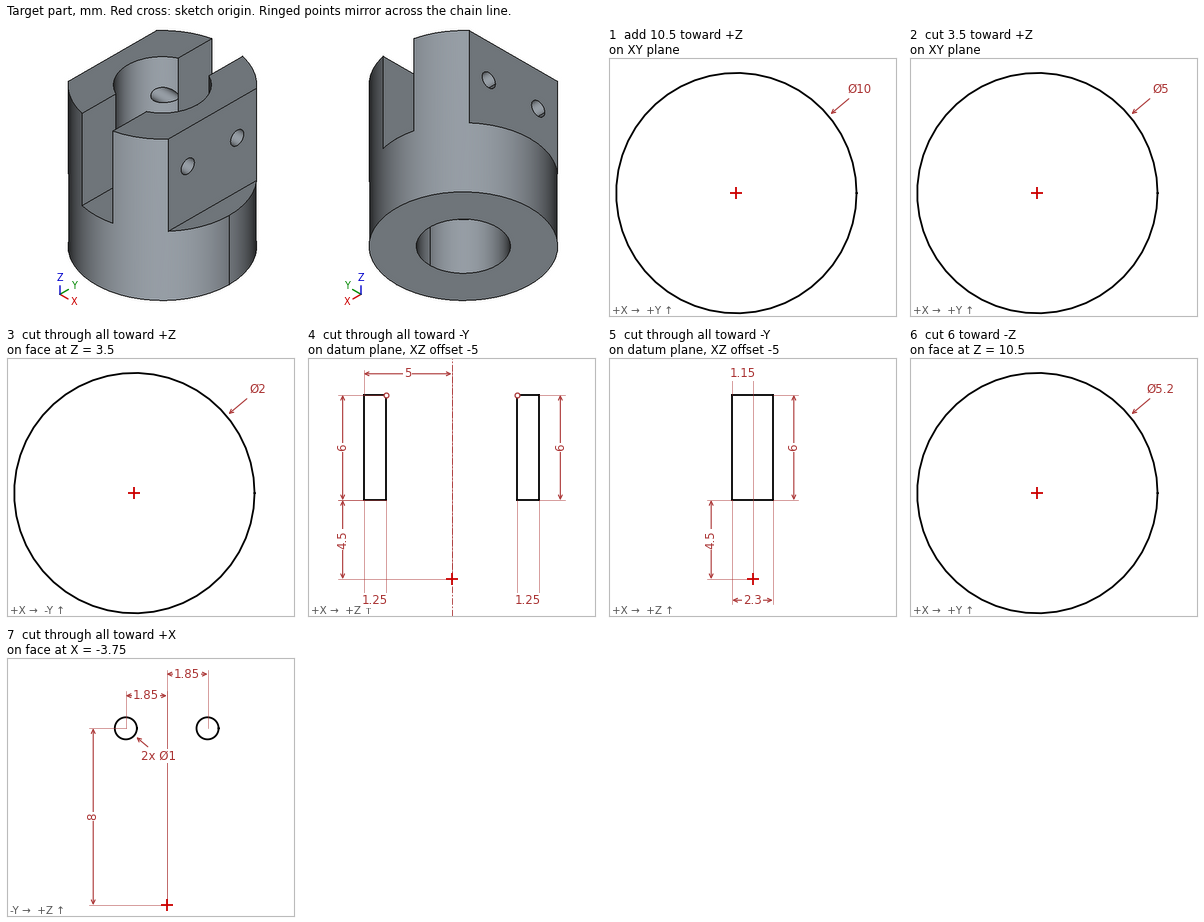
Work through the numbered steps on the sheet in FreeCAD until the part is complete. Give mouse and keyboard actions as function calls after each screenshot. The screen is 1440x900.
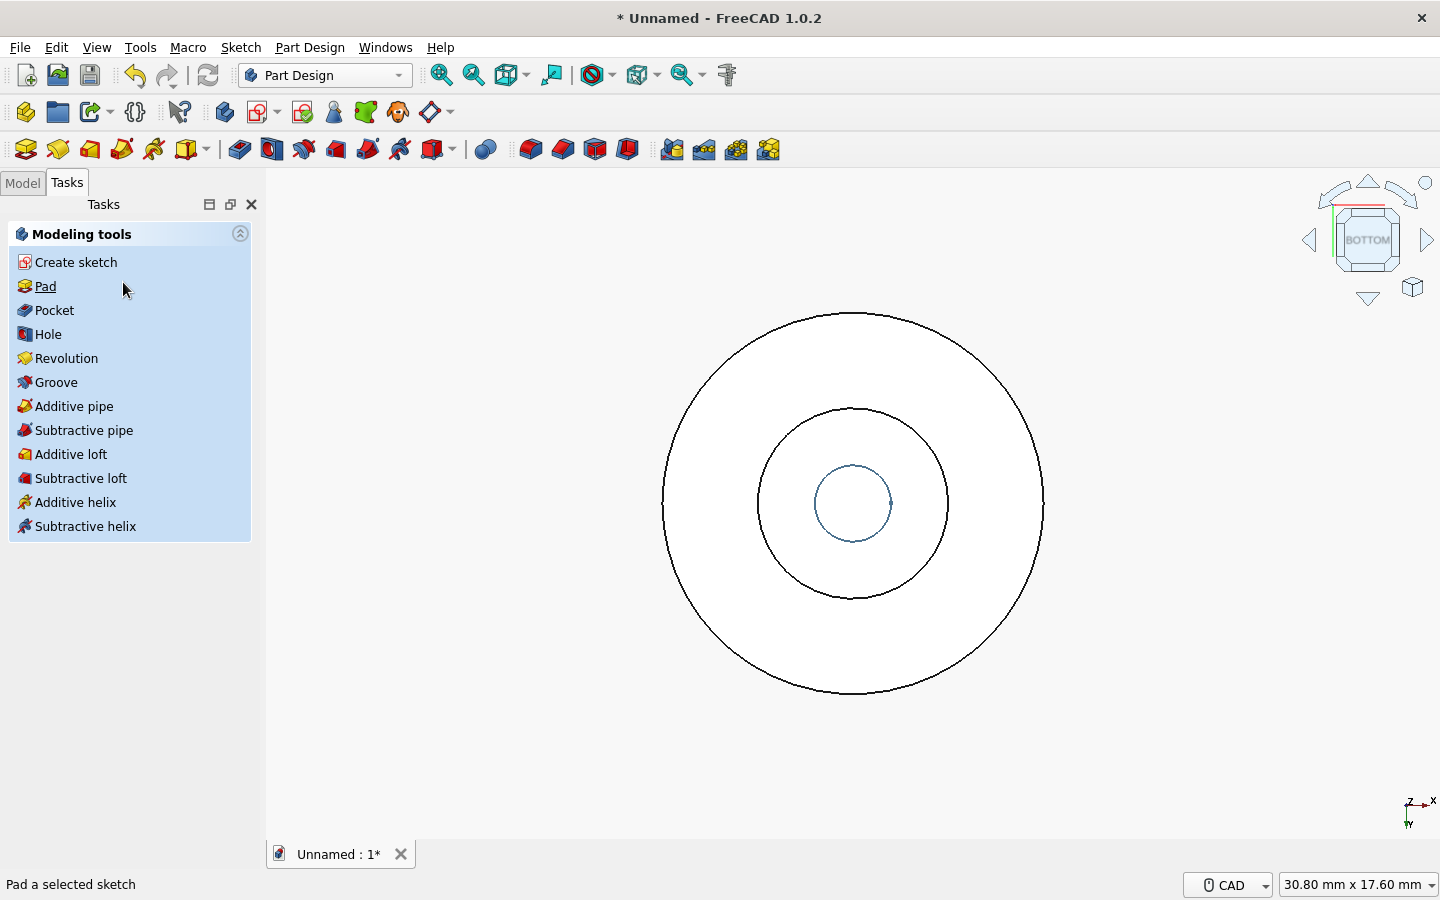
click(240, 150)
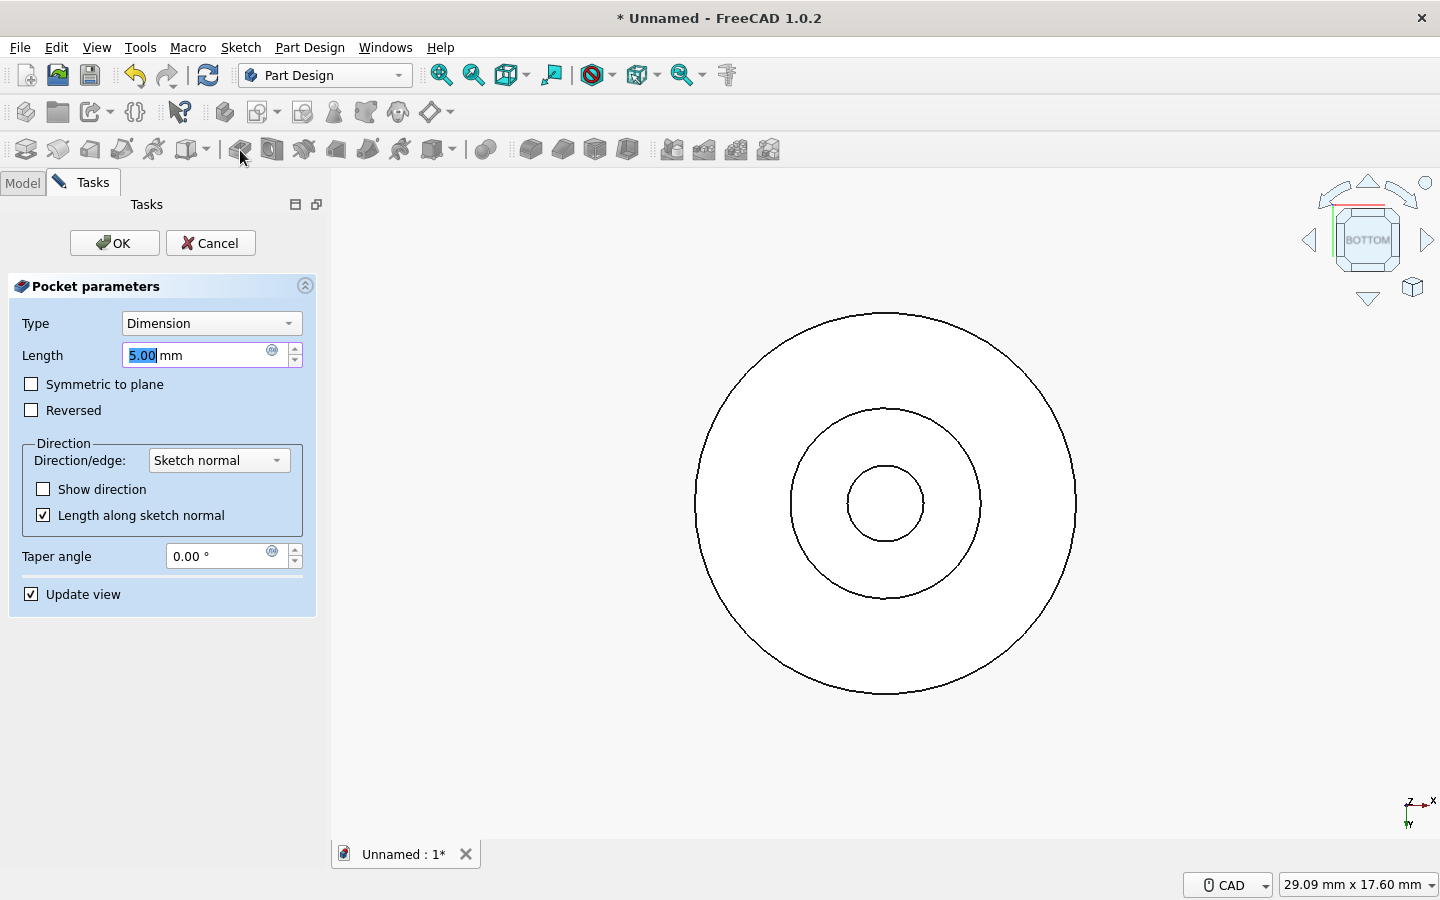
click(212, 324)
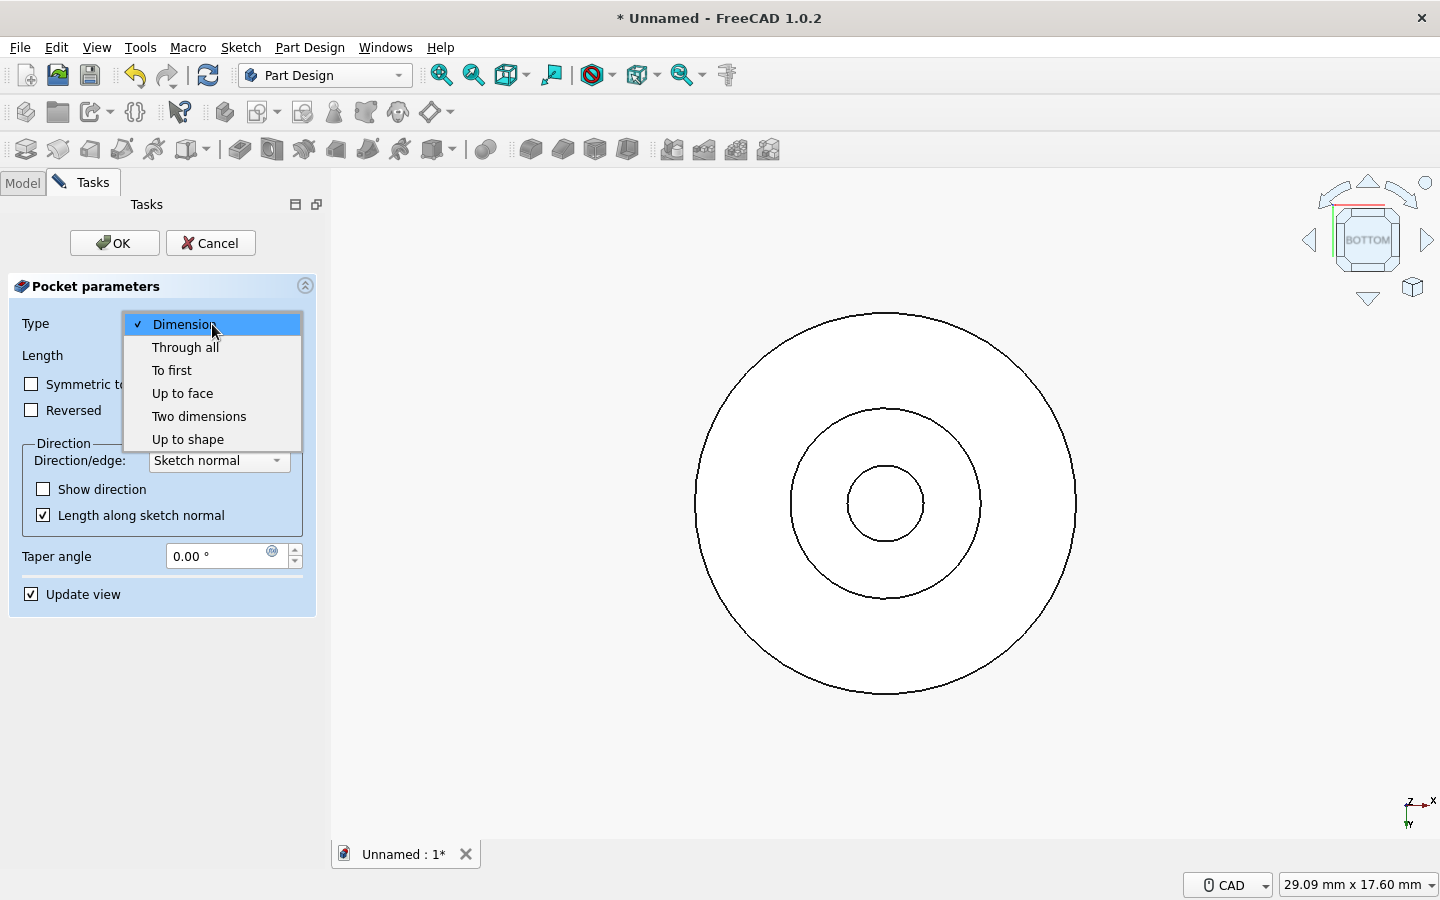
click(212, 348)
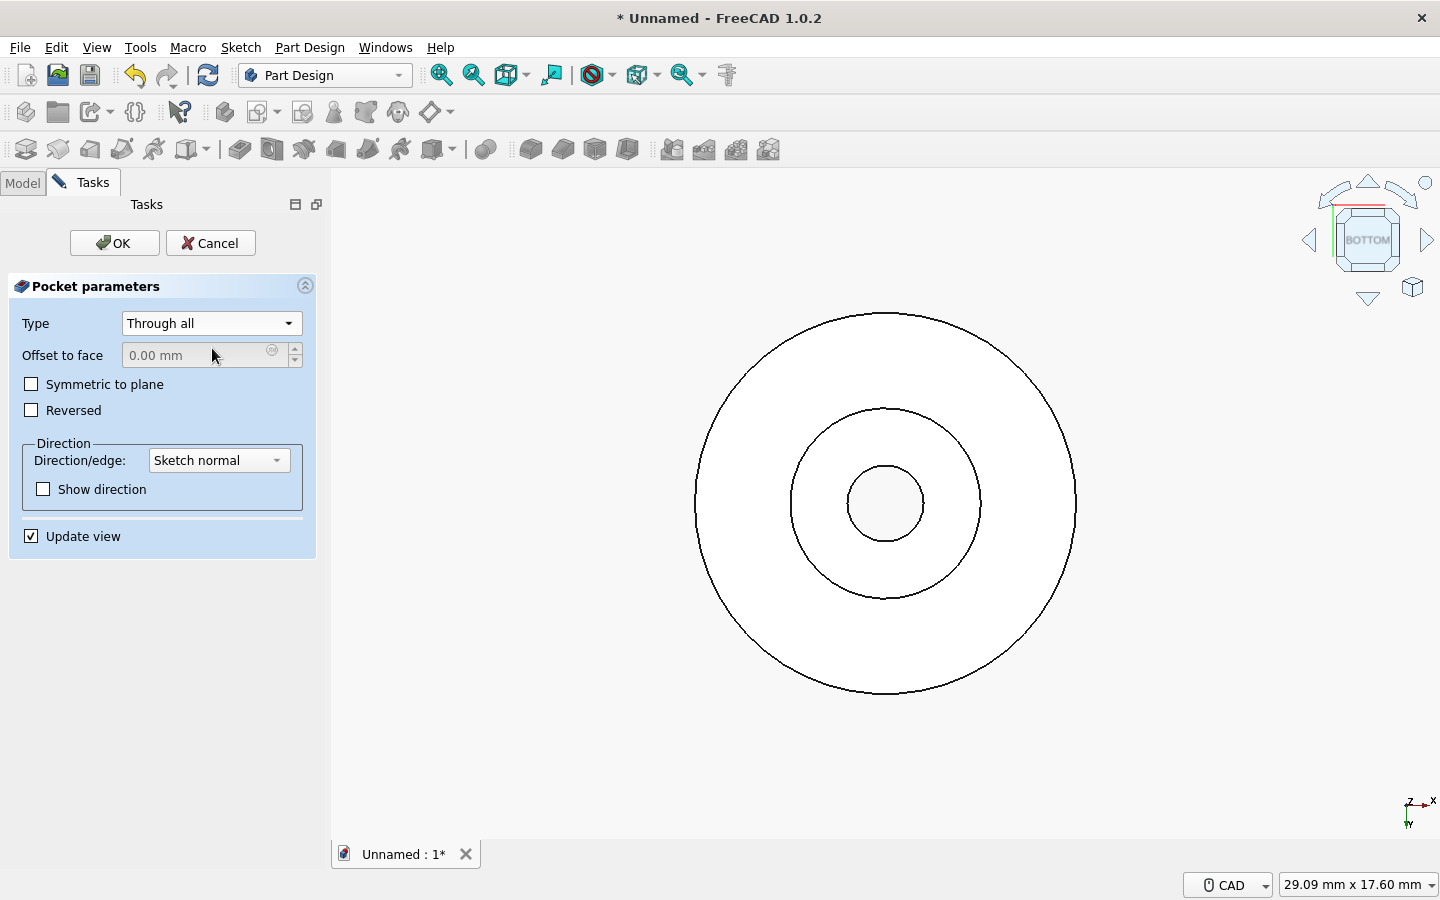
click(115, 243)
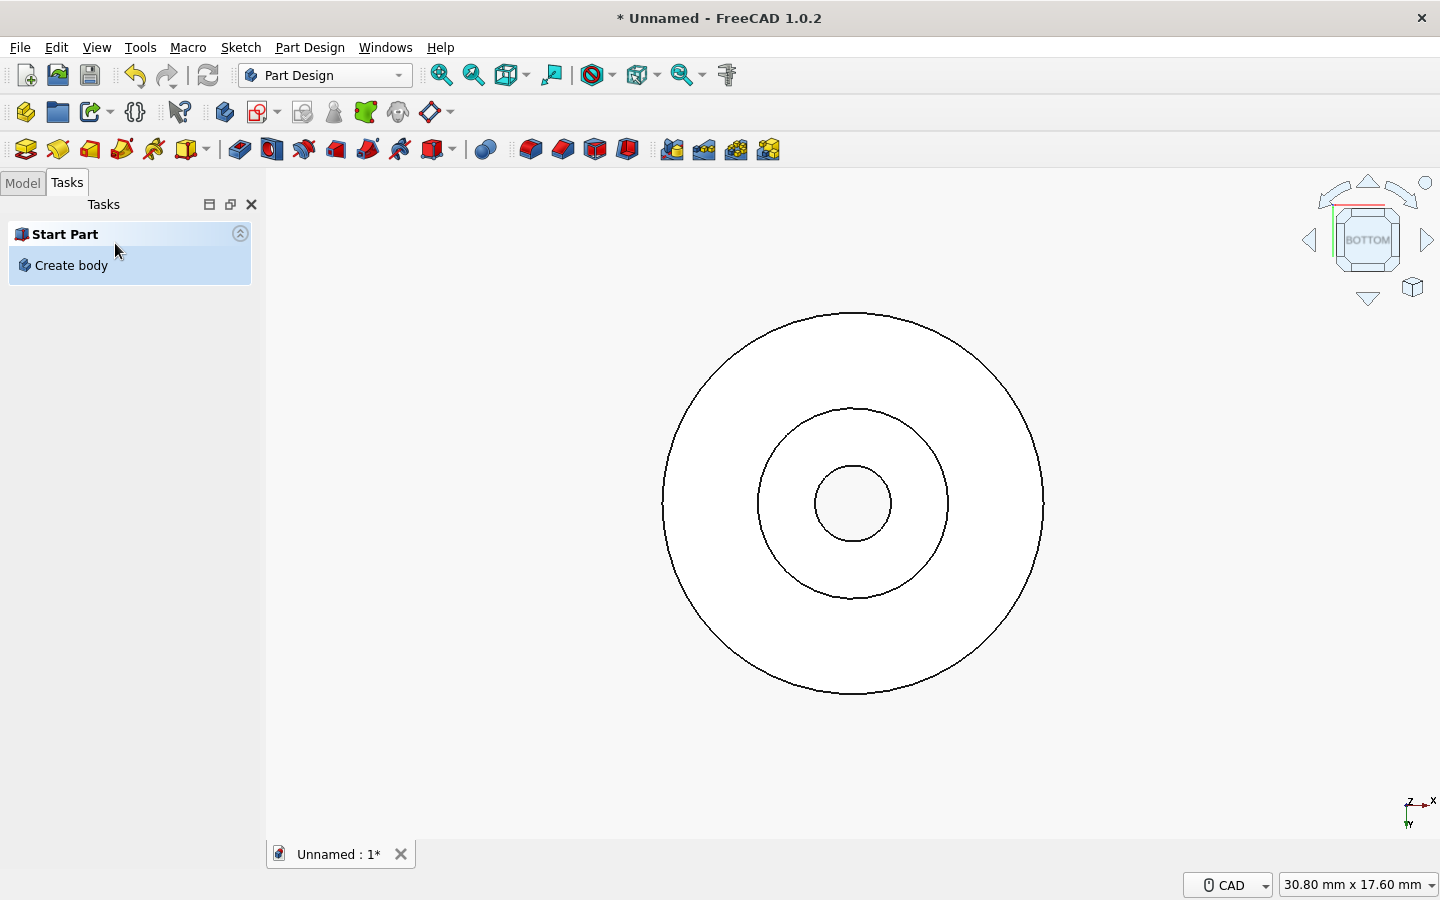
click(23, 182)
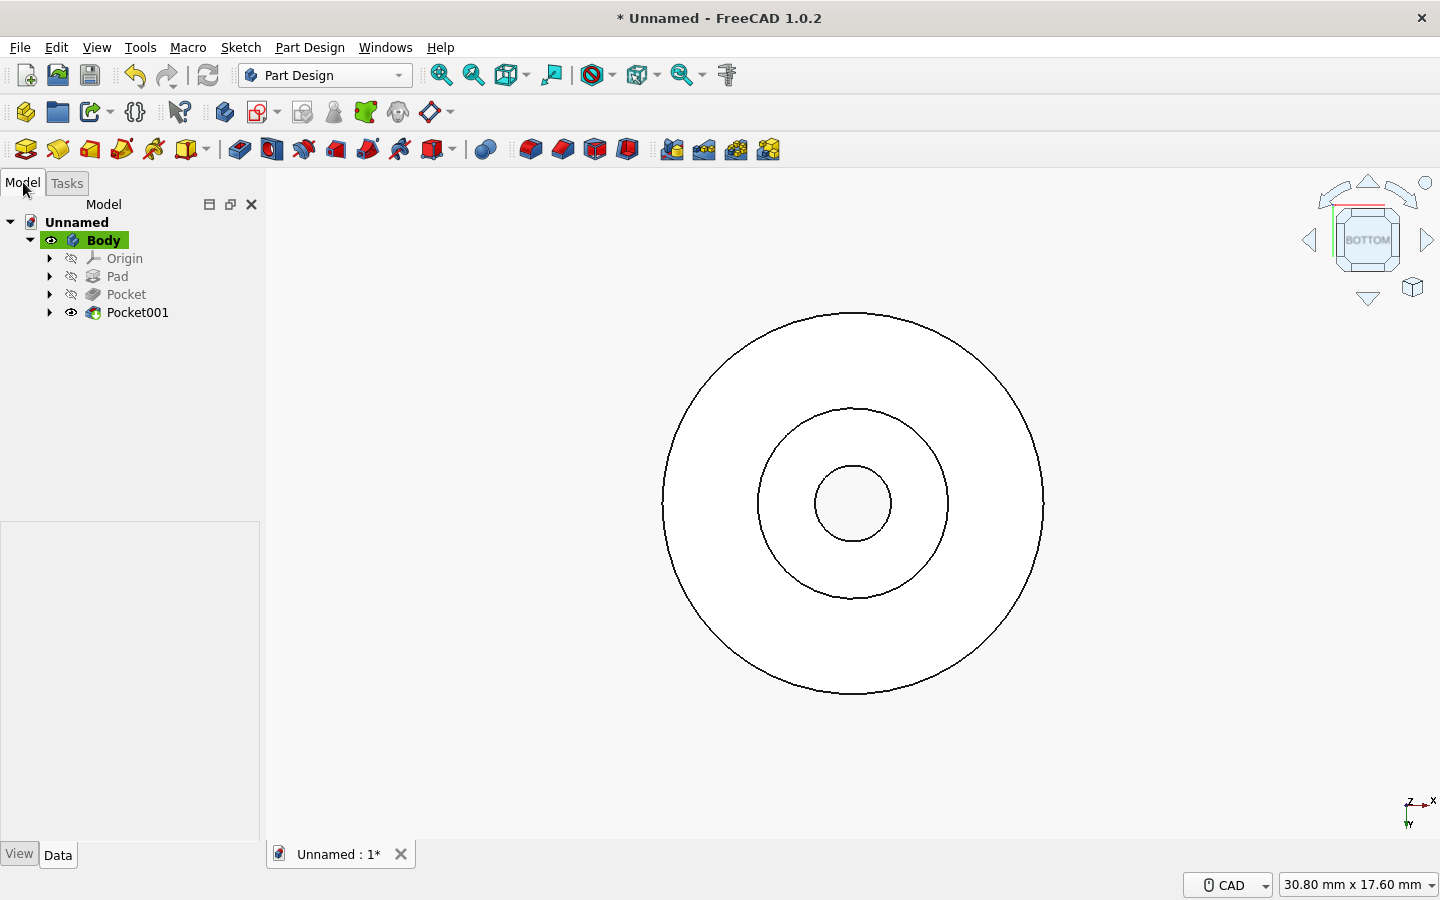
click(50, 258)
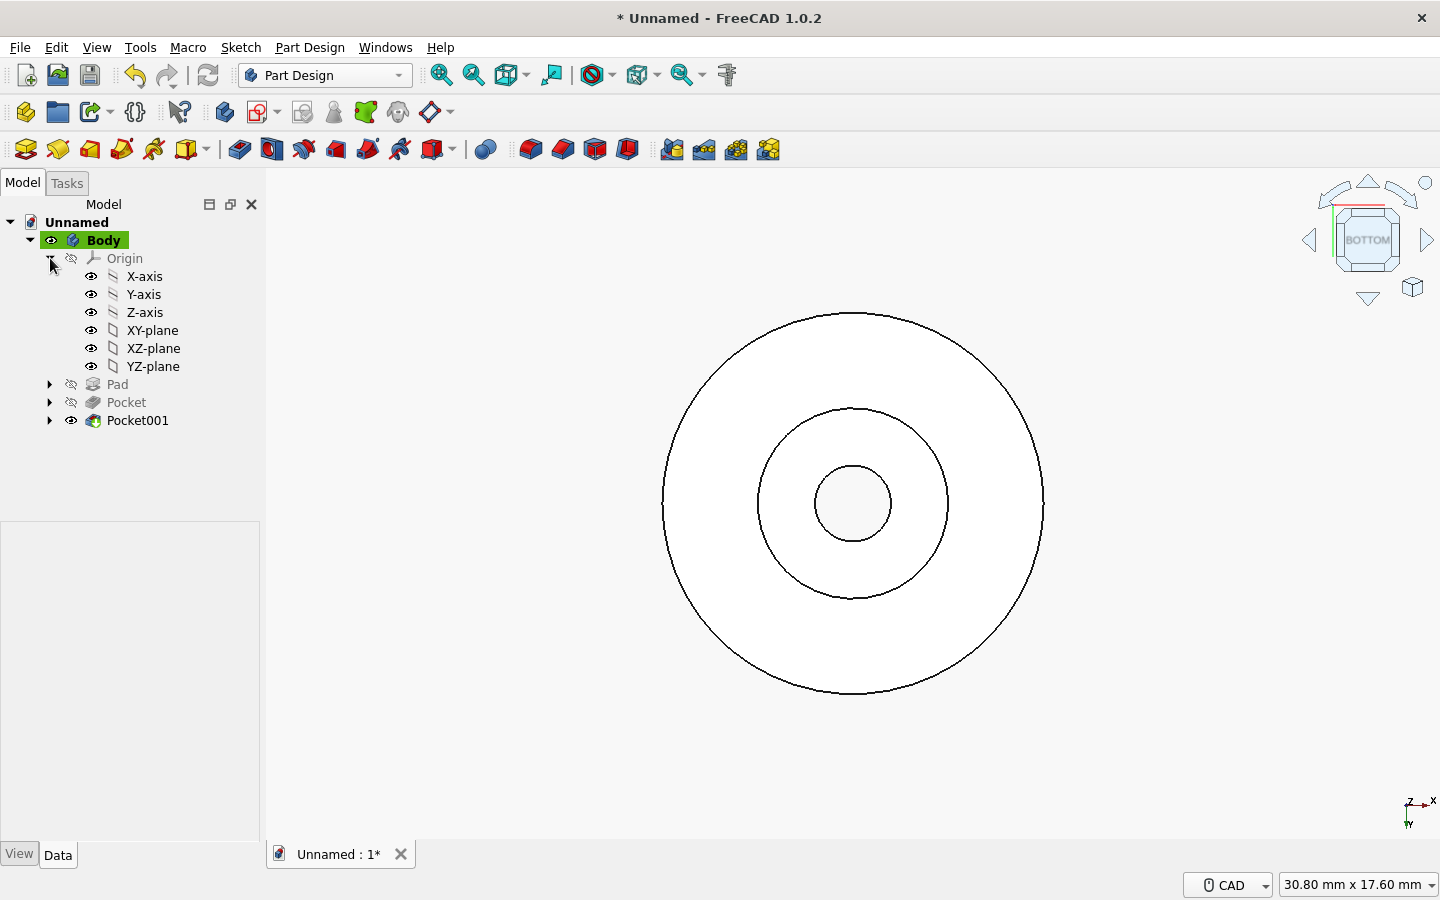
click(136, 348)